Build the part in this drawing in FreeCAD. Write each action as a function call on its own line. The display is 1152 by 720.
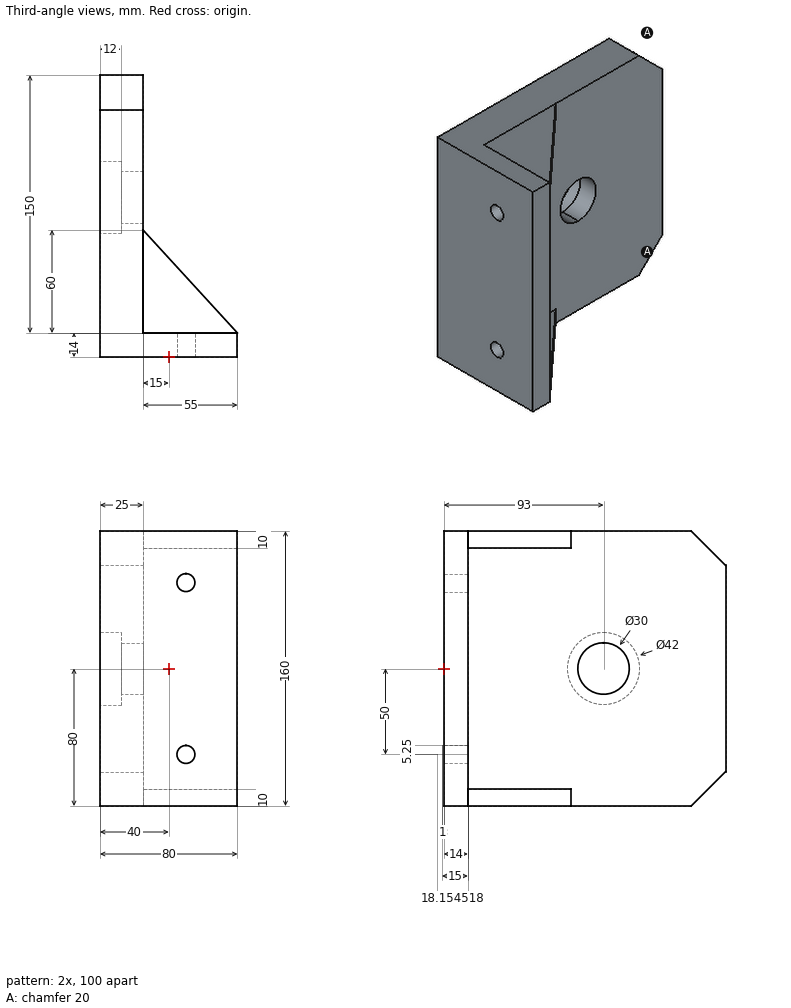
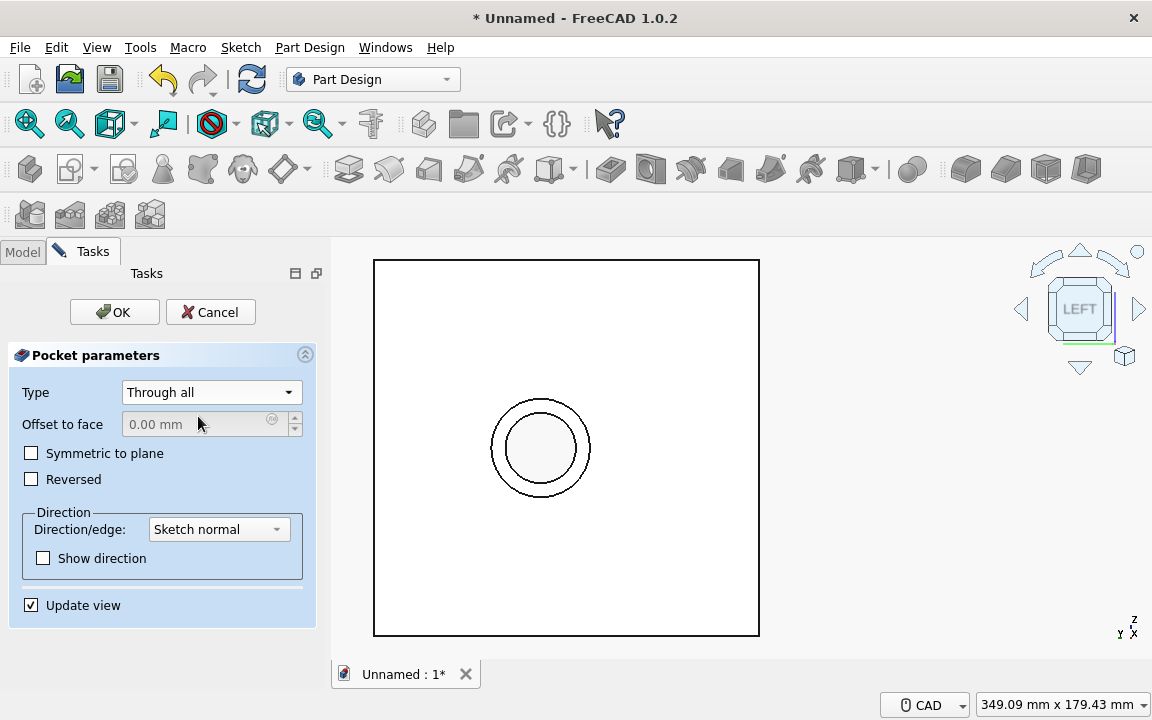
click(115, 312)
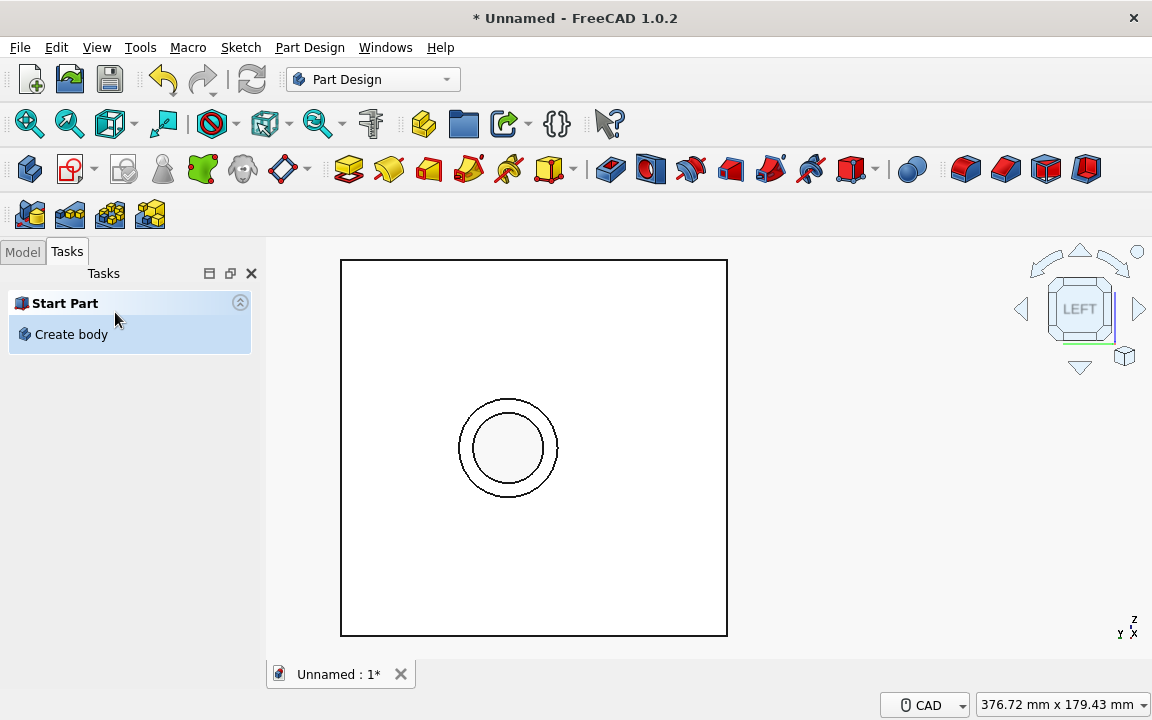
click(23, 251)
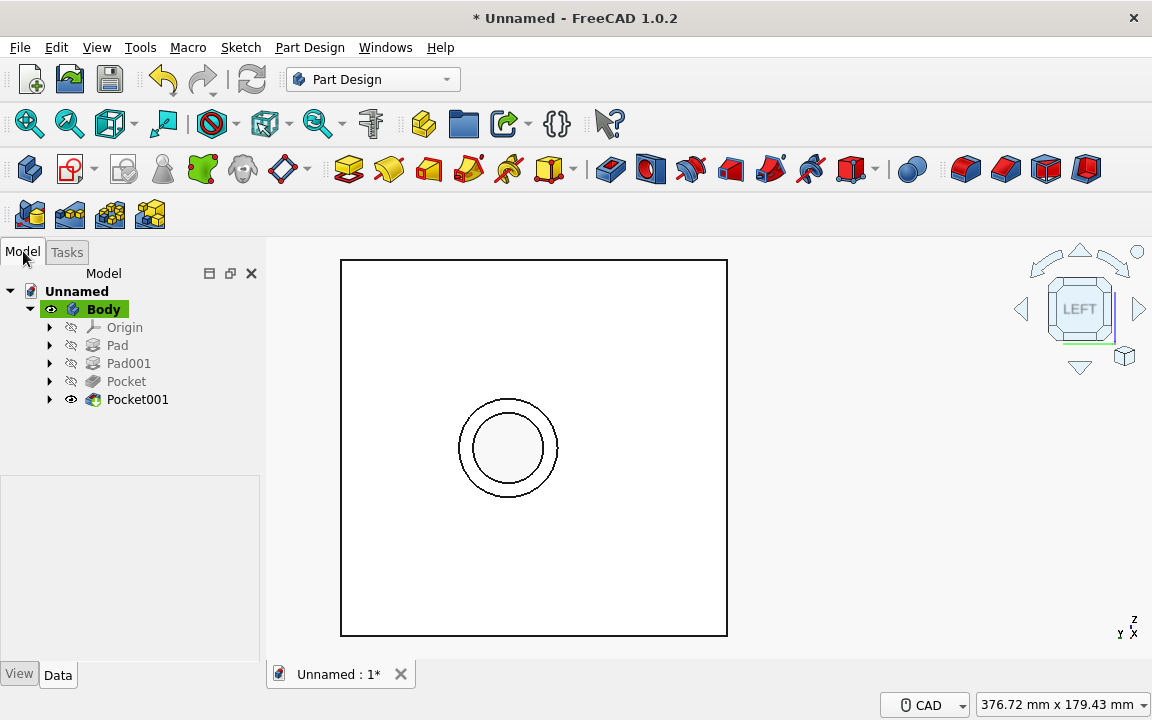
click(50, 327)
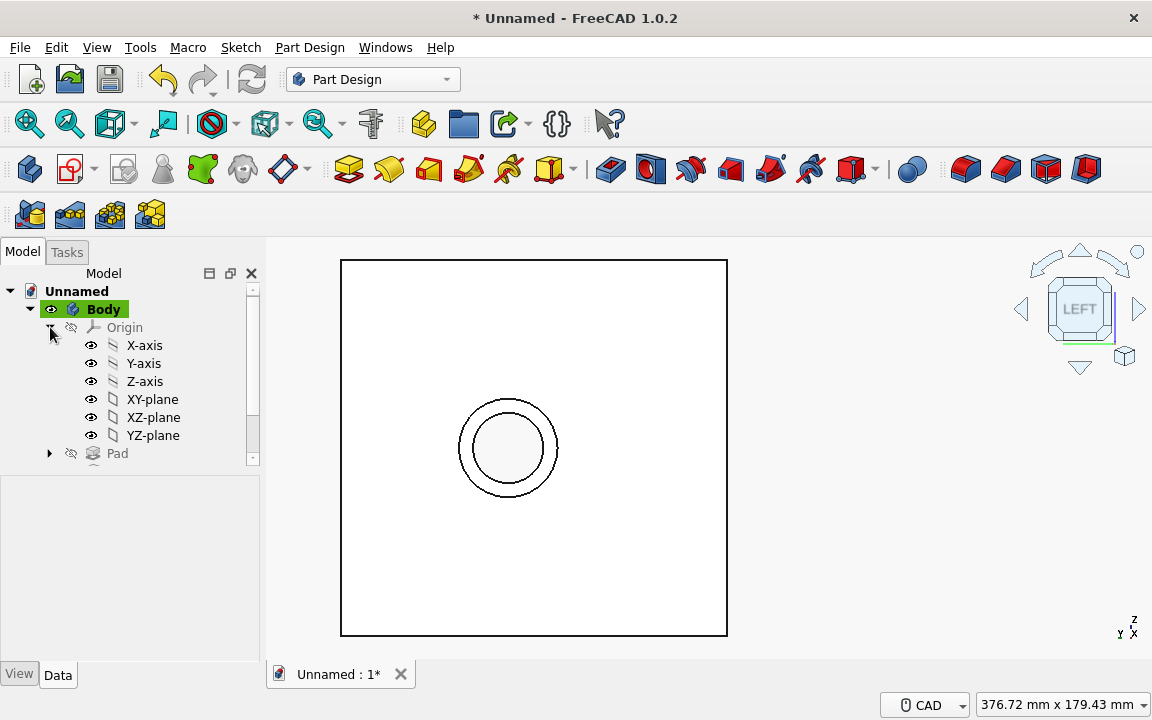
click(136, 435)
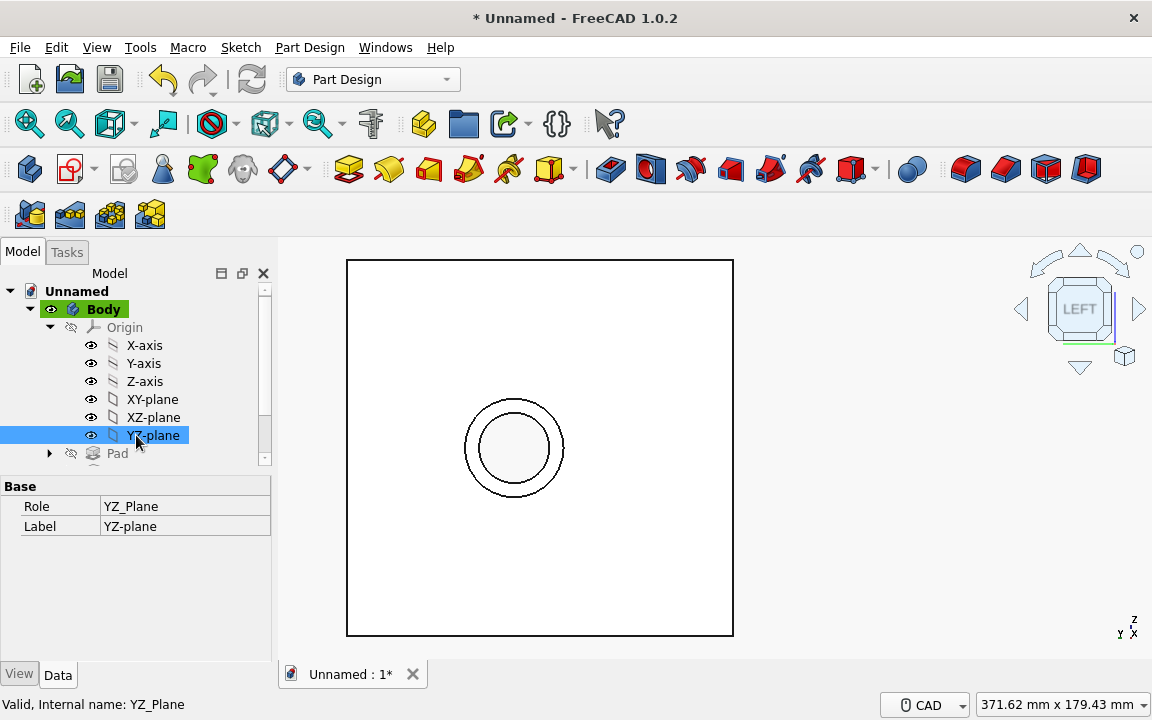
click(284, 170)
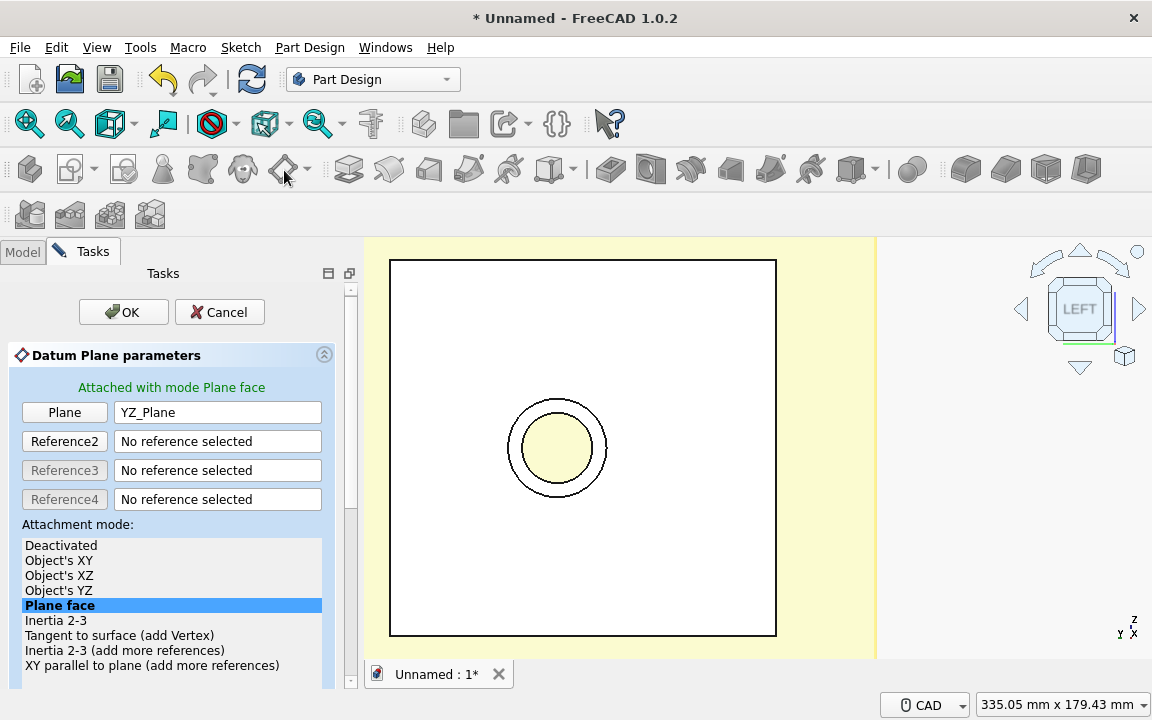
scroll(351, 486, down, 4)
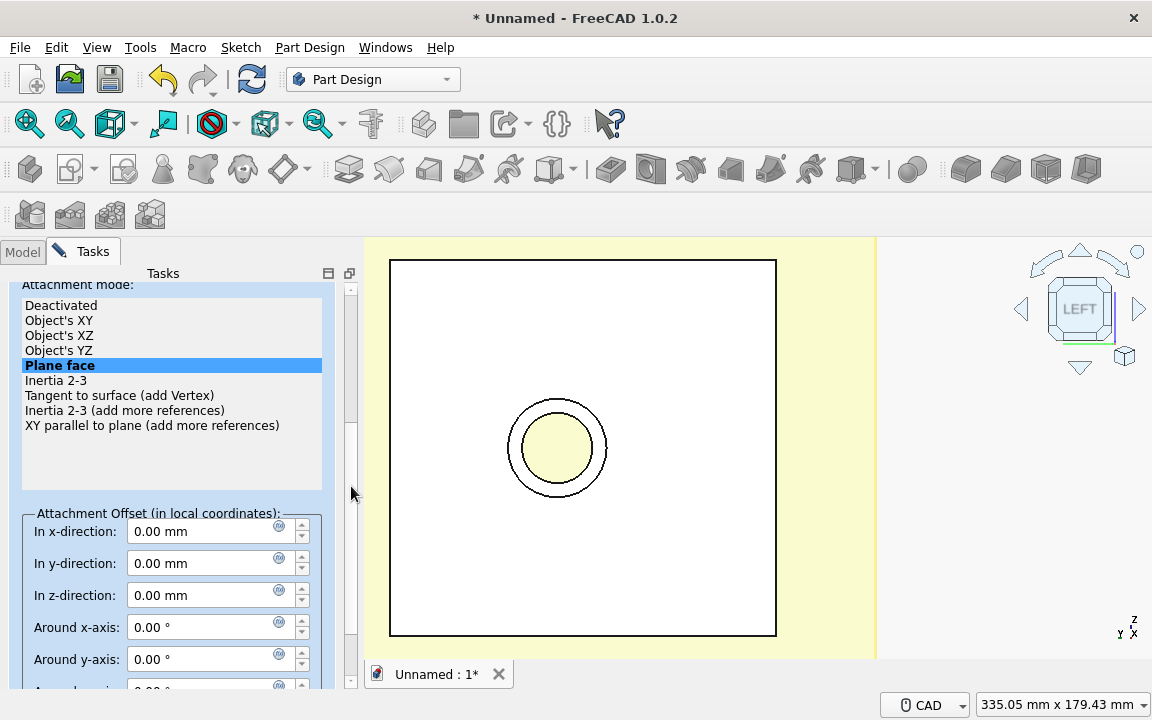
triple_click(210, 595)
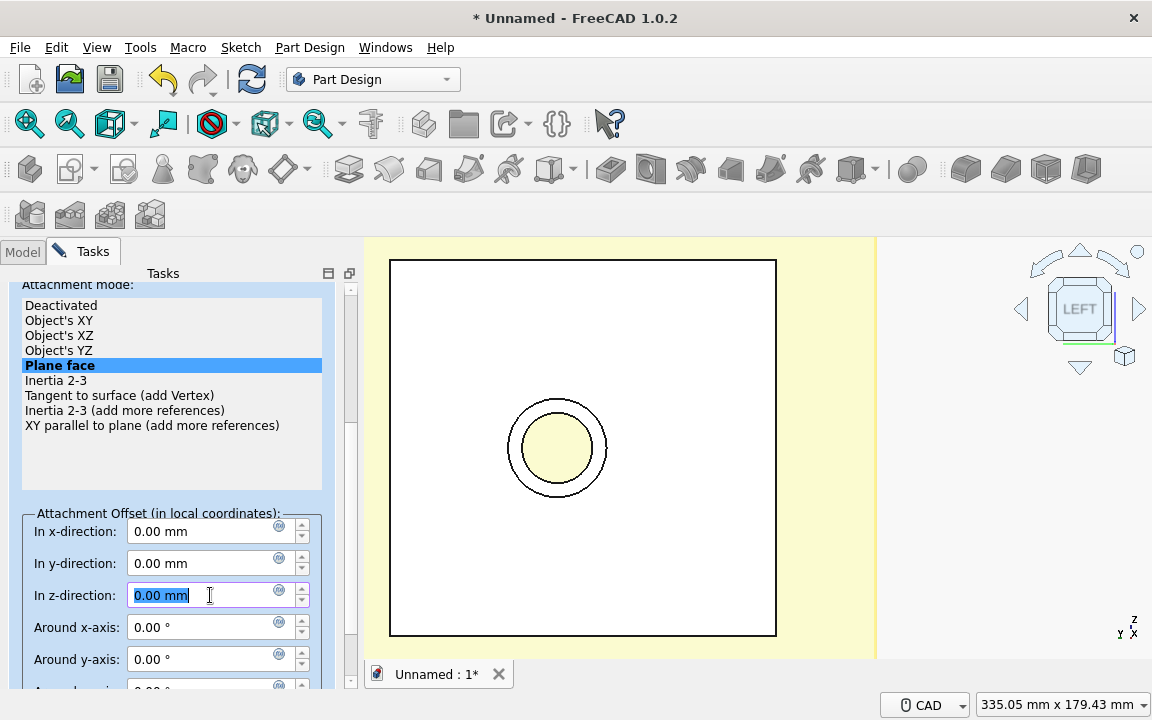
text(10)
key(Tab)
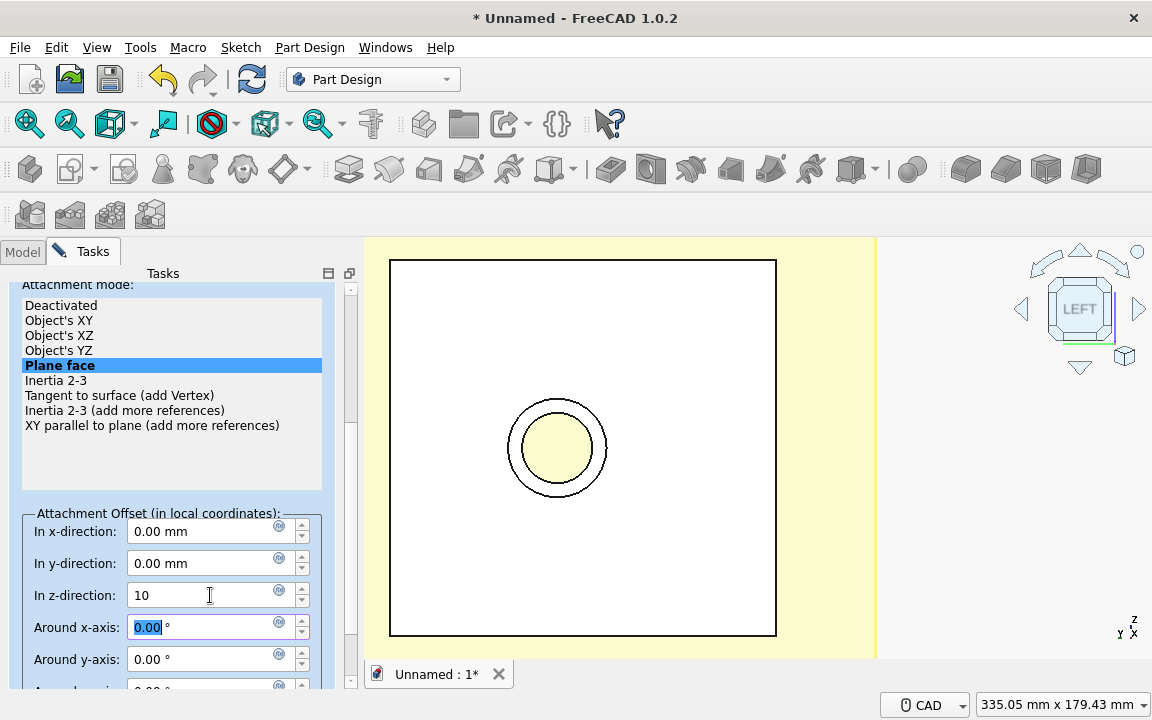
scroll(351, 486, up, 5)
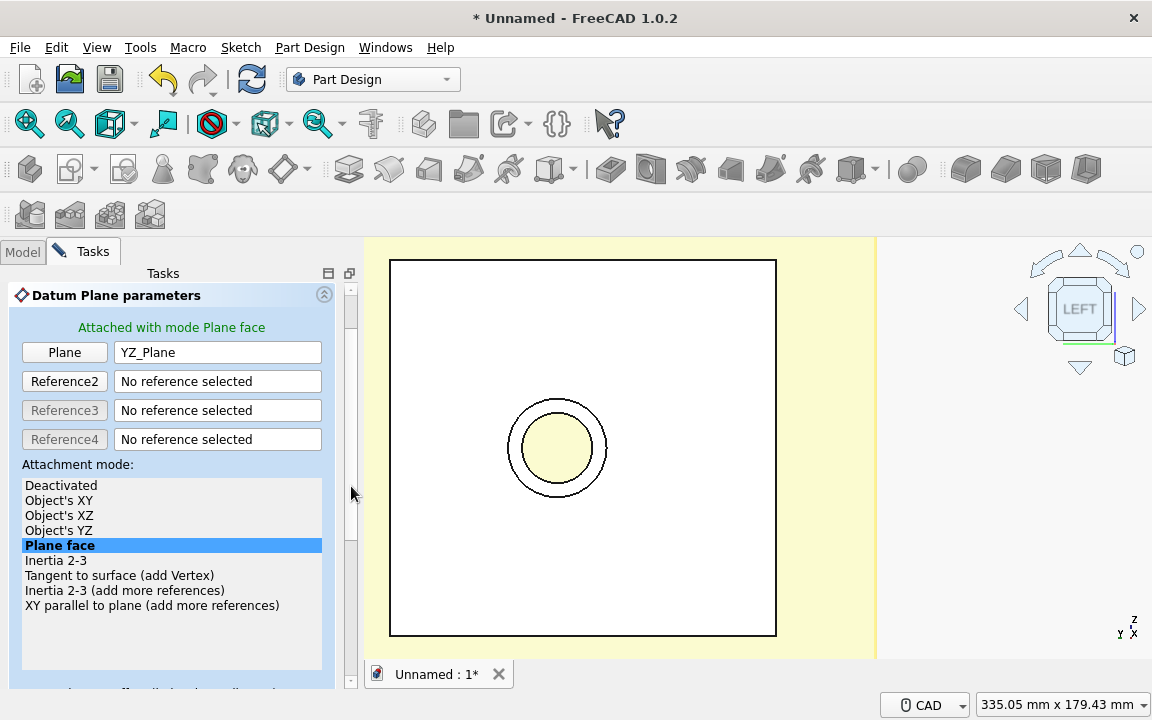
click(124, 312)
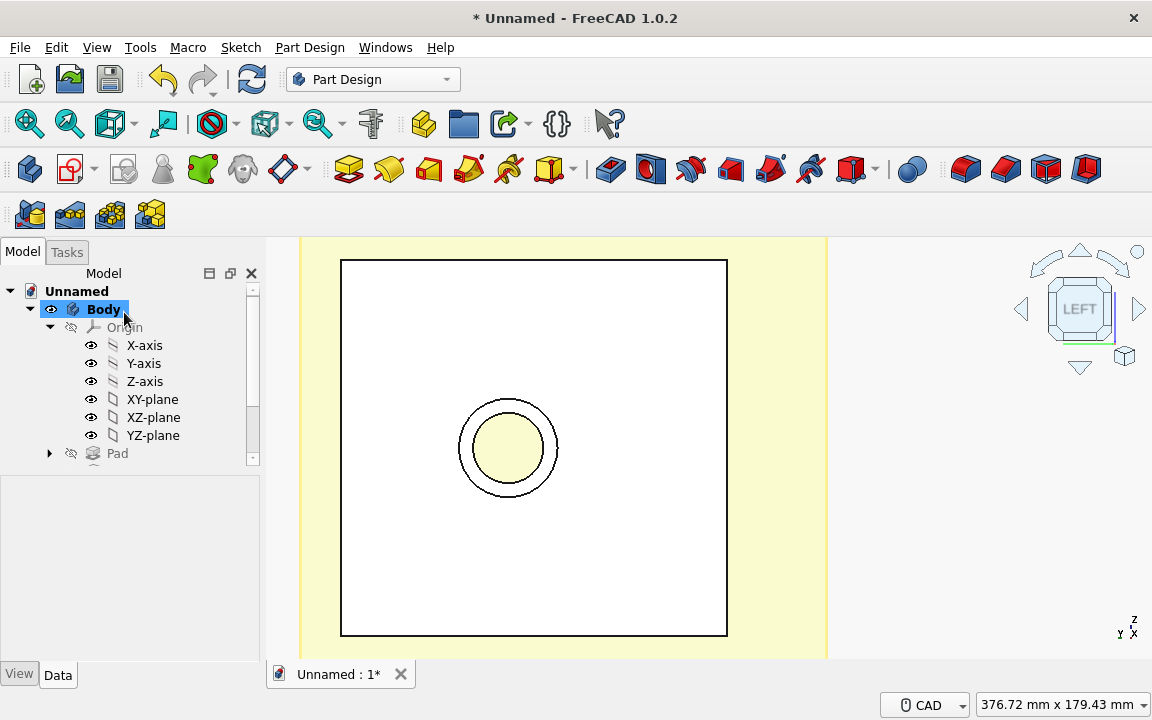
scroll(100, 377, down, 3)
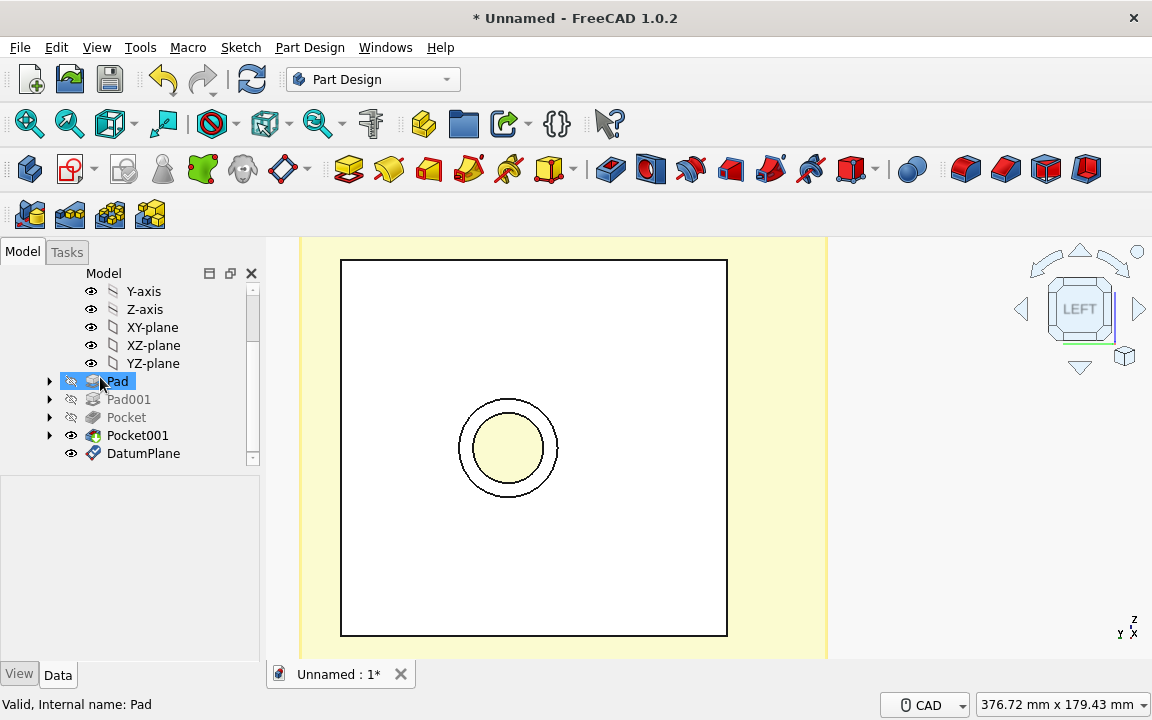
click(116, 453)